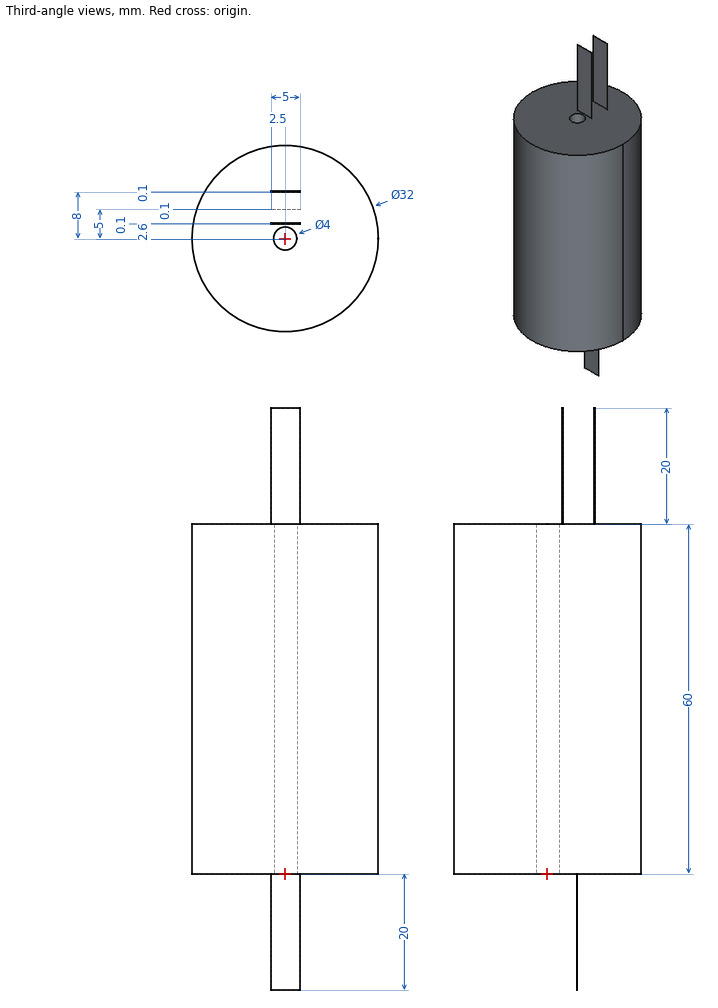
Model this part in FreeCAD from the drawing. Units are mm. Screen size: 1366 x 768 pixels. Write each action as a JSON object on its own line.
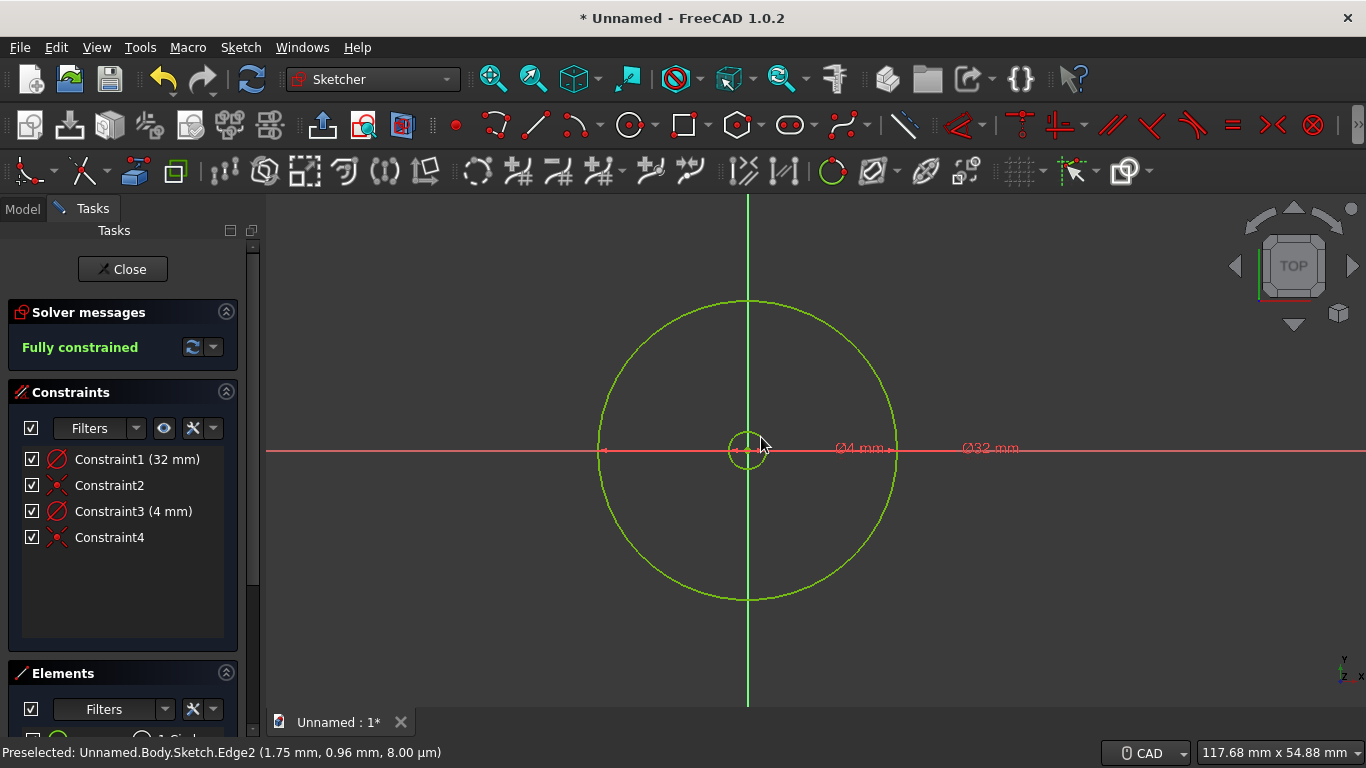
{"action": "left_click", "coordinate": [123, 269]}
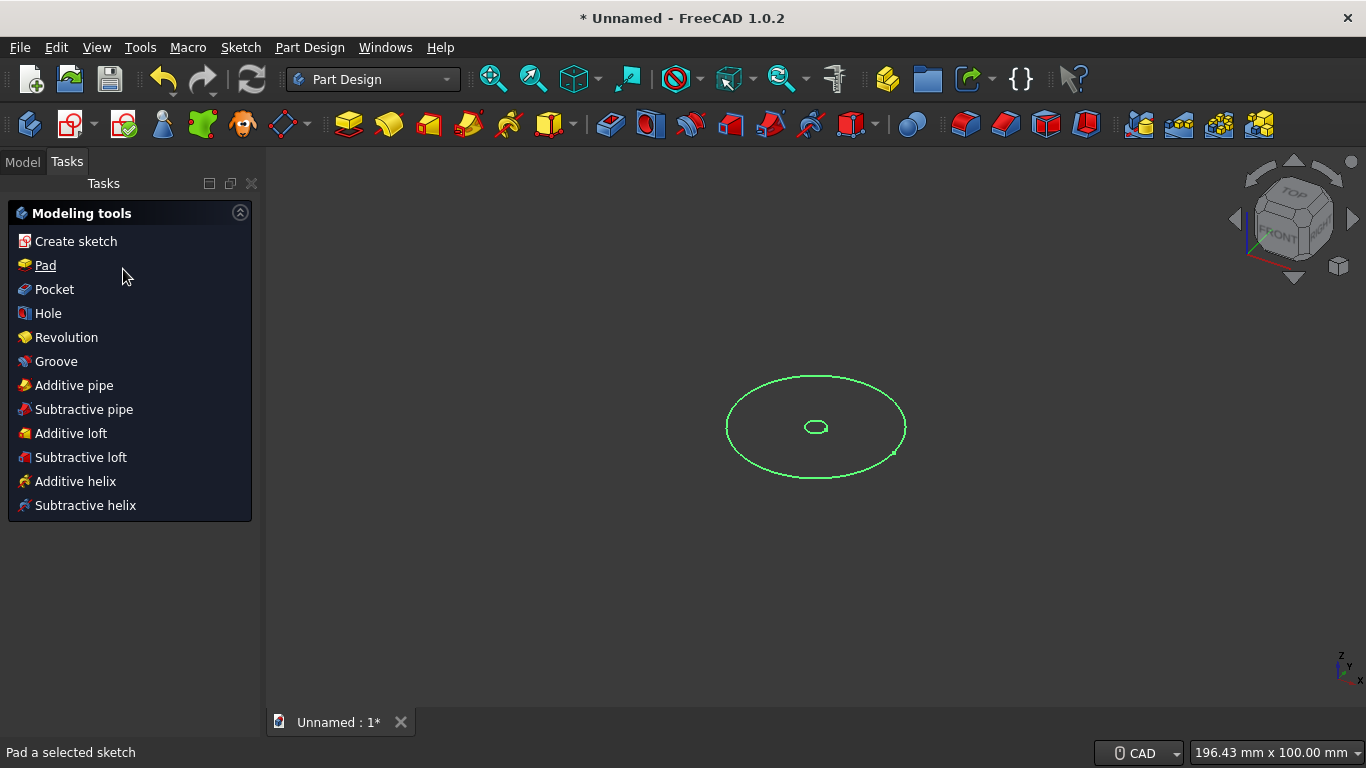
{"action": "left_click", "coordinate": [350, 124]}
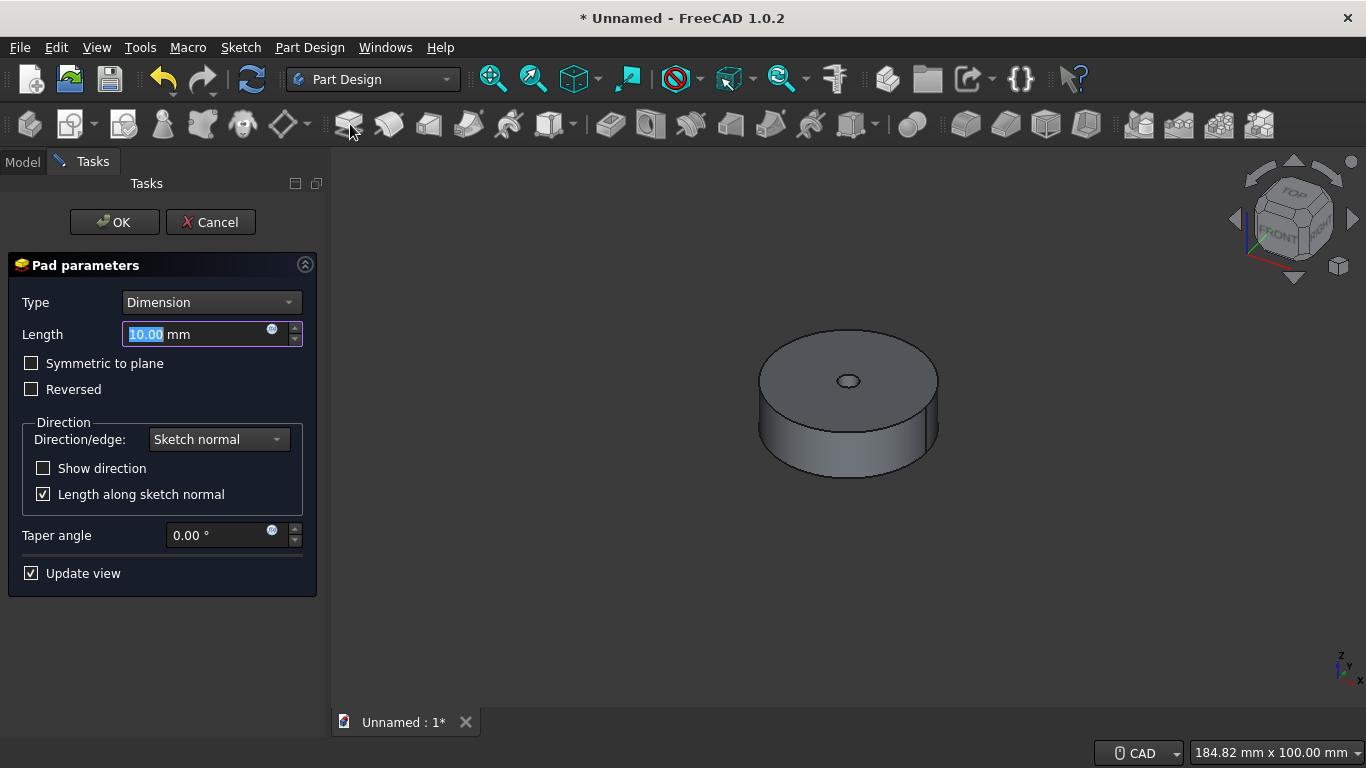
{"action": "type", "text": "60"}
{"action": "key", "text": "Tab"}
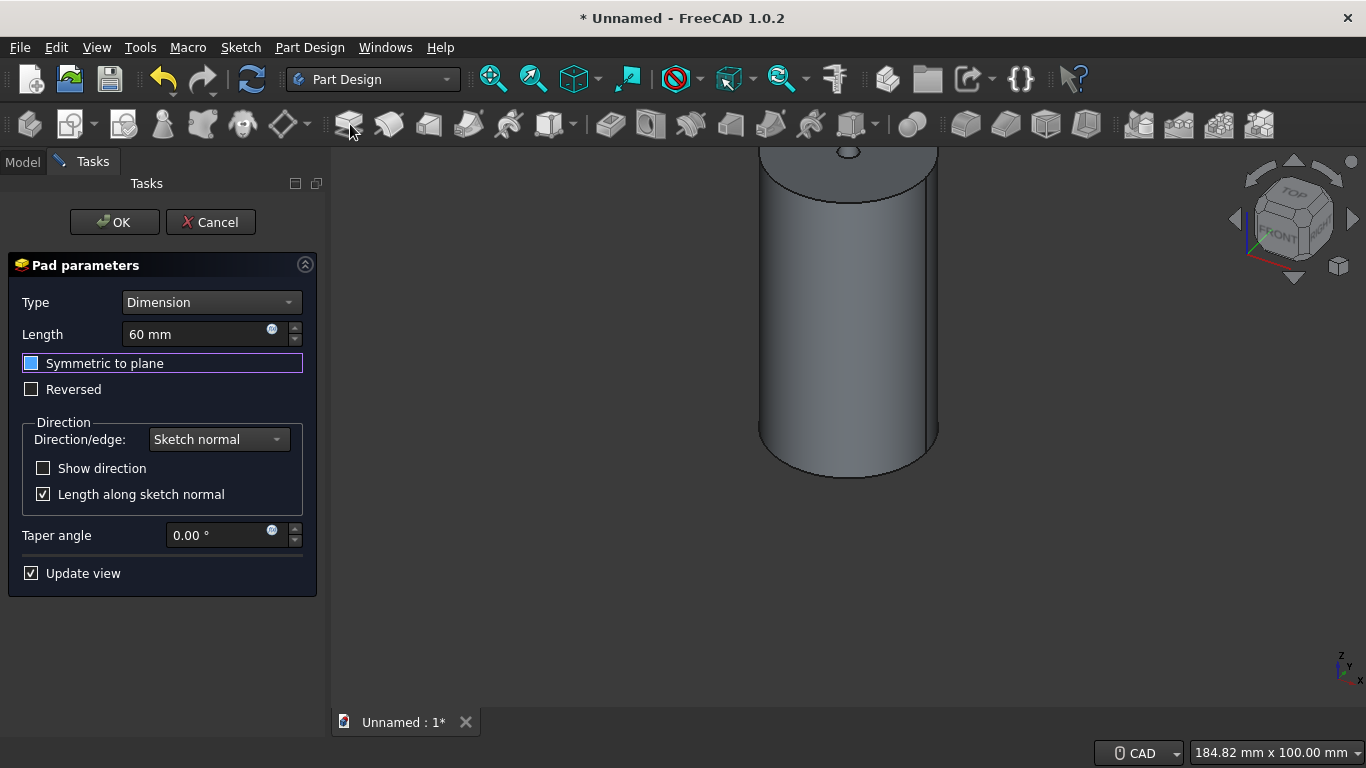
{"action": "left_click", "coordinate": [115, 222]}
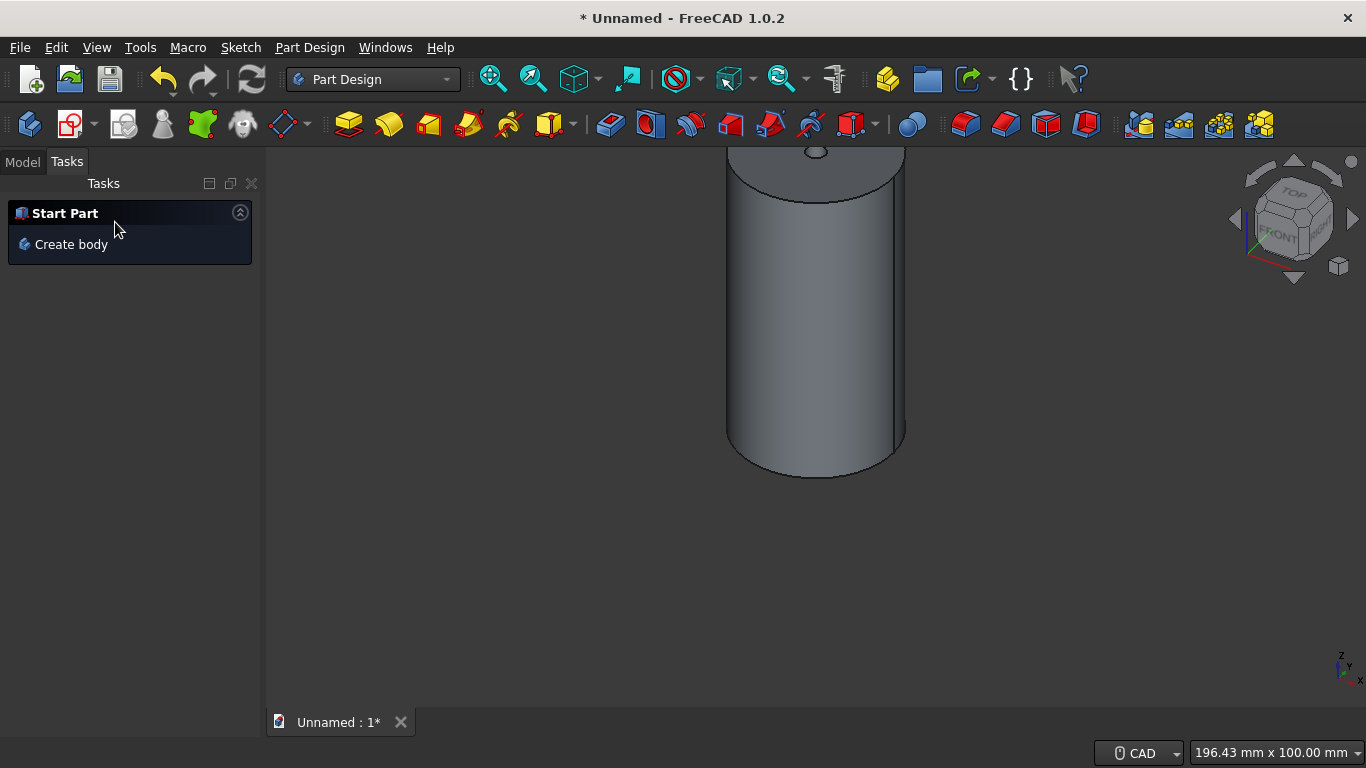
{"action": "left_click", "coordinate": [494, 80]}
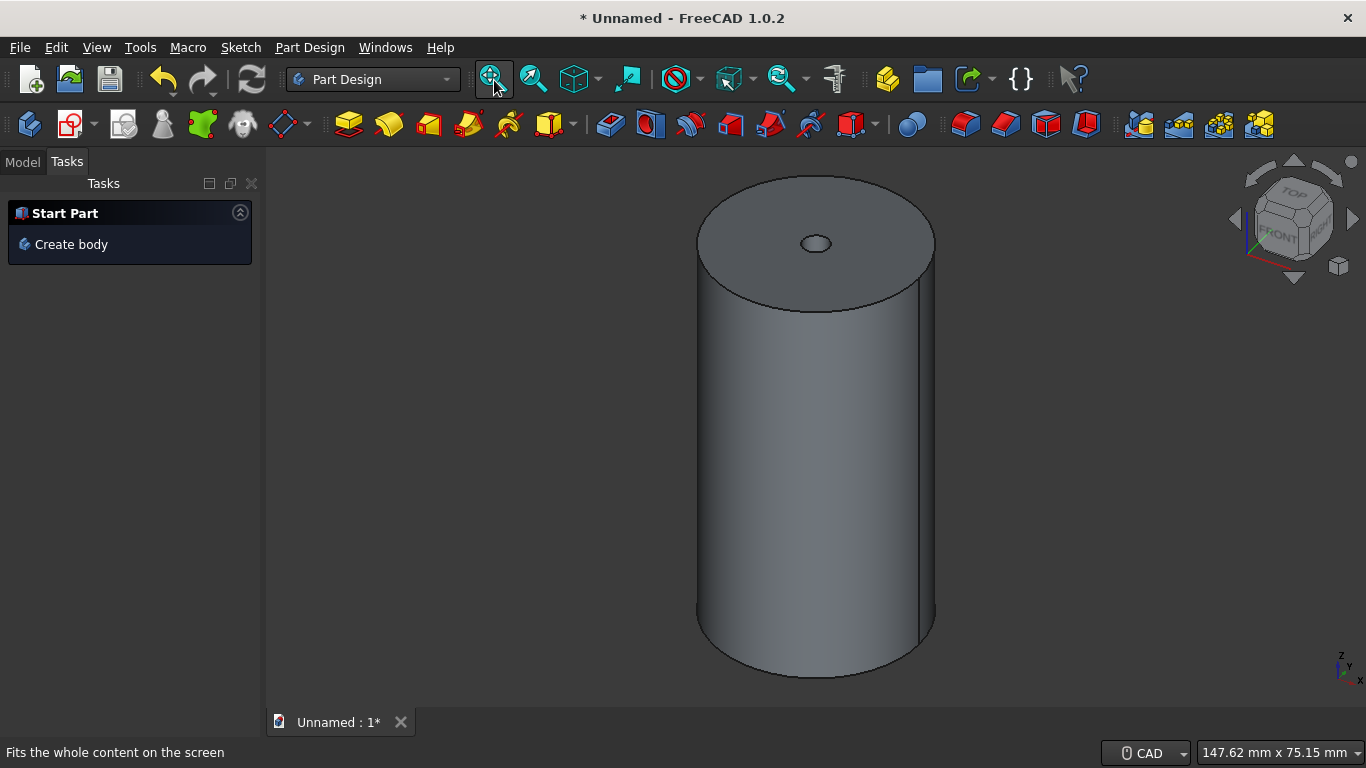
{"action": "key", "text": "5"}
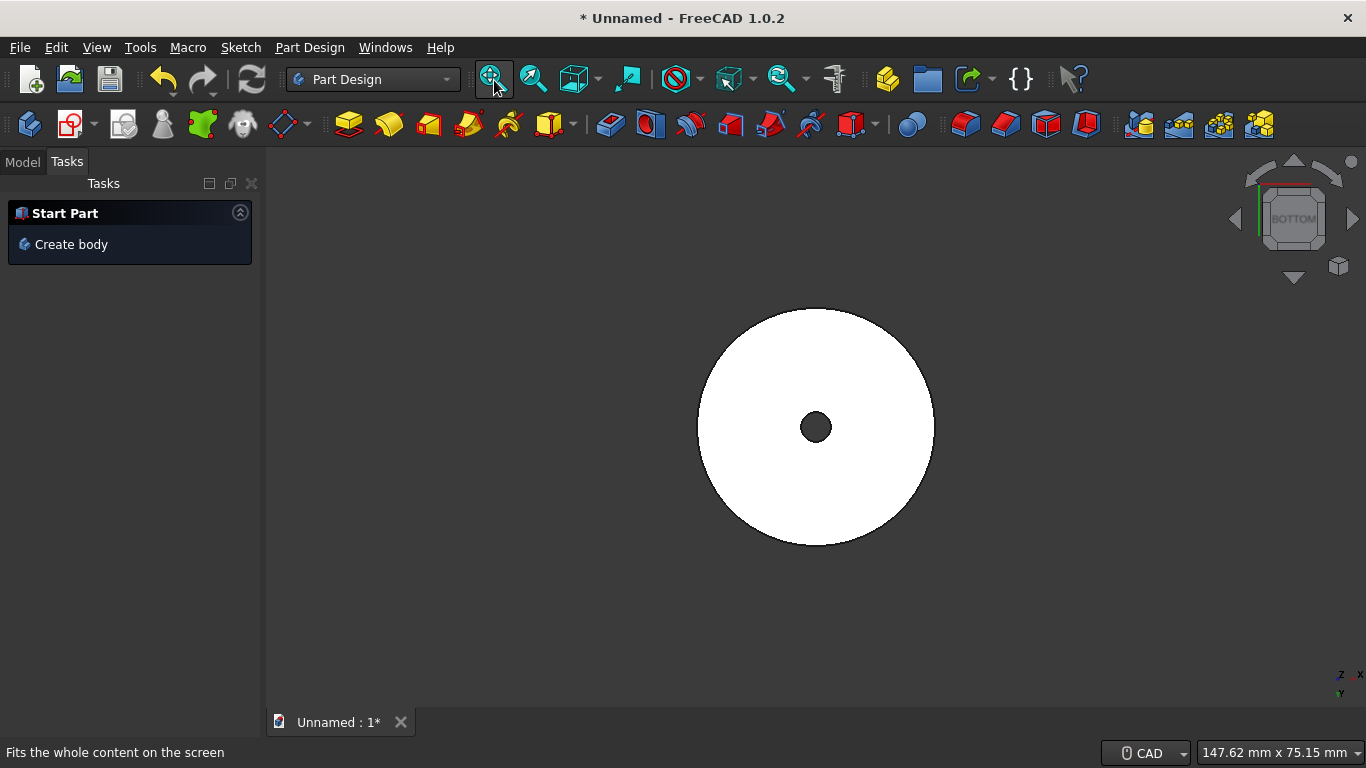
{"action": "left_click", "coordinate": [494, 80]}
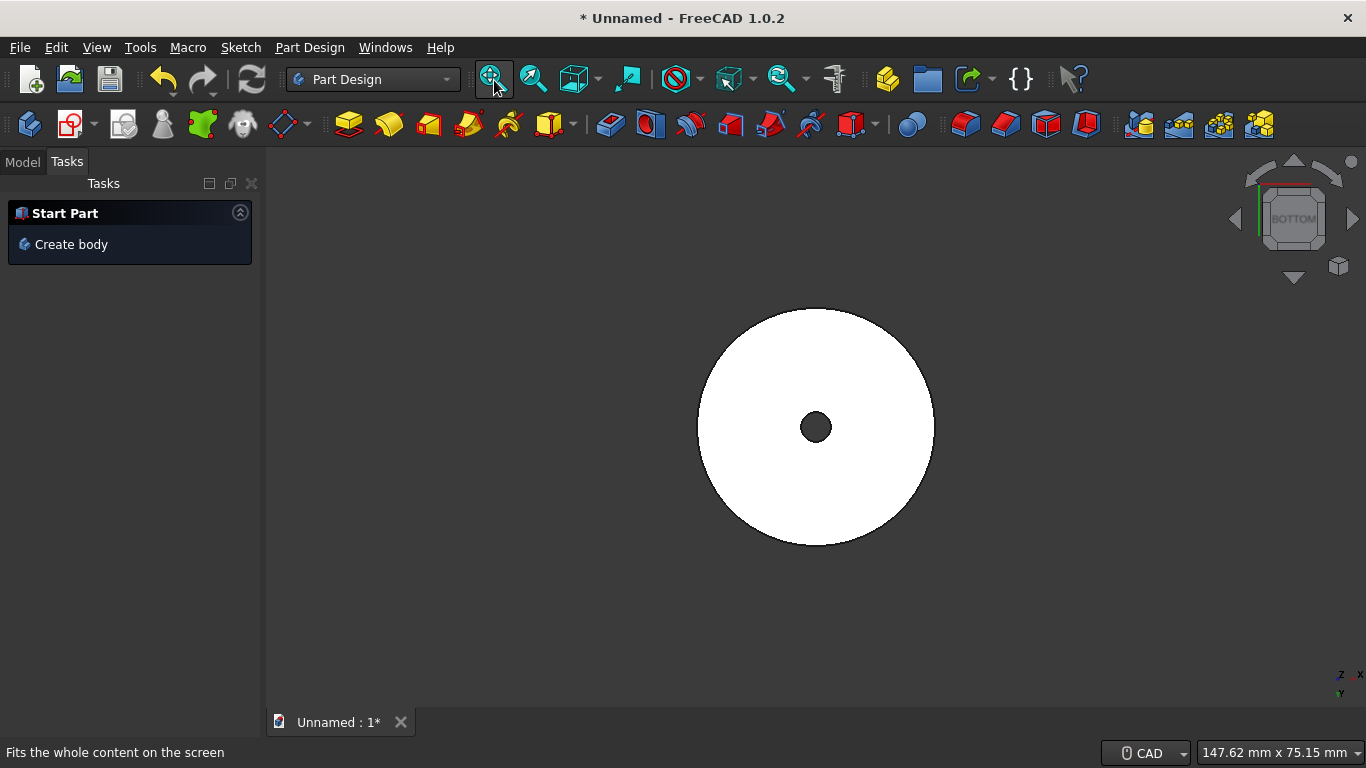
{"action": "left_click", "coordinate": [816, 358]}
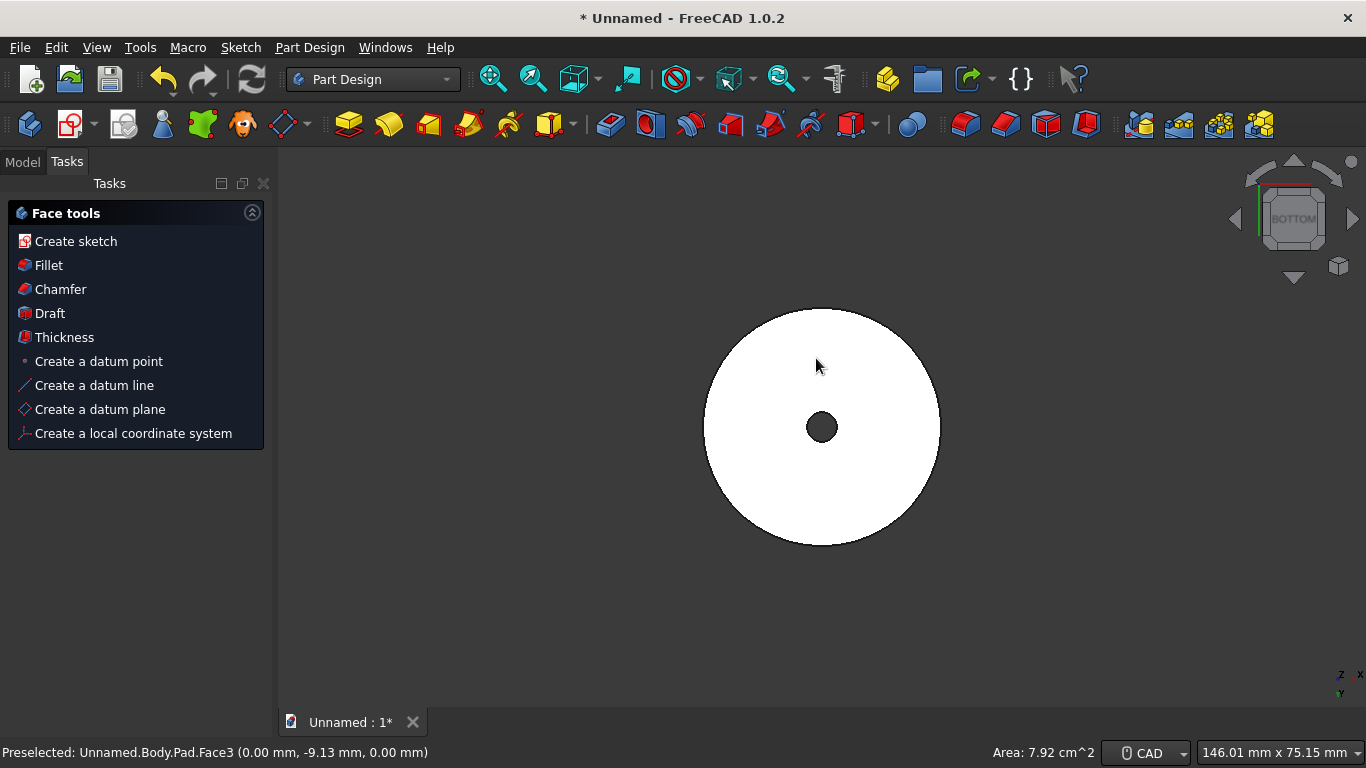
{"action": "left_click", "coordinate": [70, 124]}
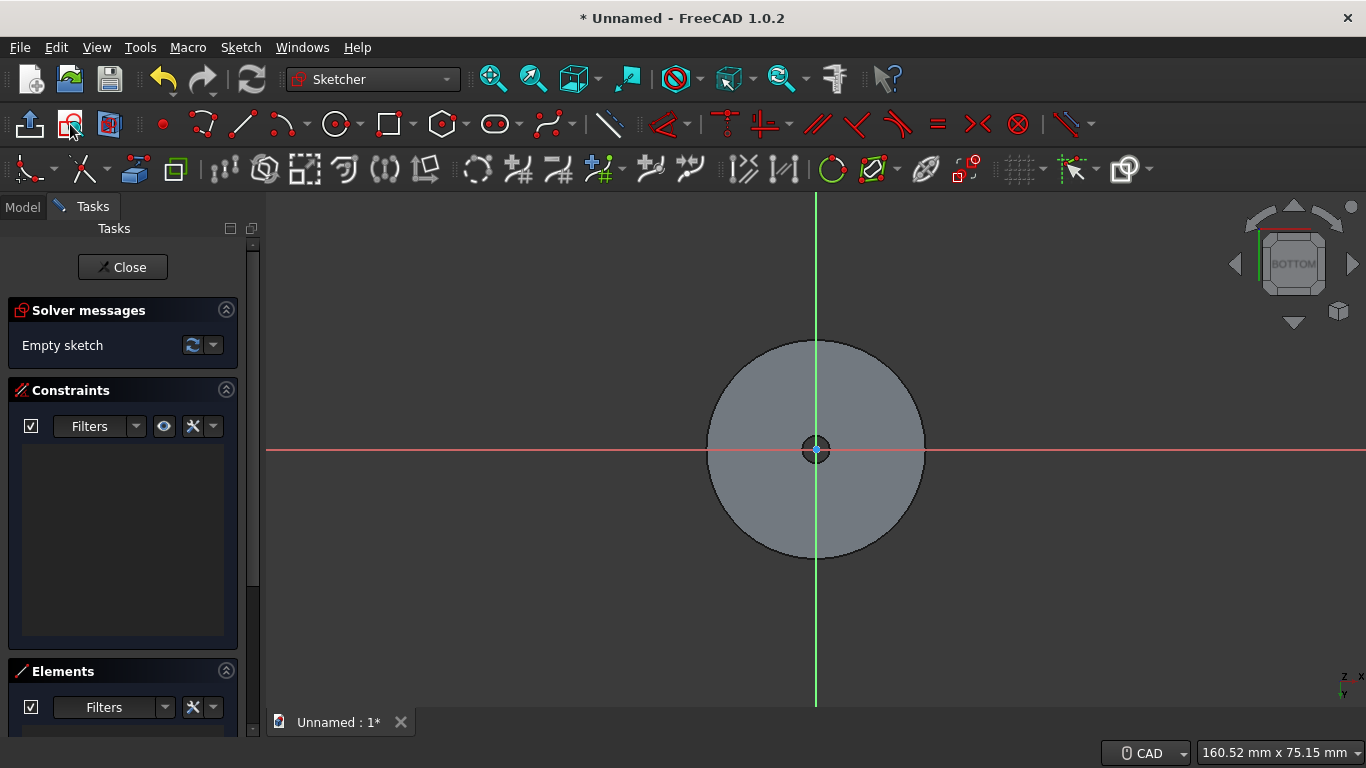
{"action": "scroll", "coordinate": [825, 469], "scroll_direction": "up", "scroll_amount": 11}